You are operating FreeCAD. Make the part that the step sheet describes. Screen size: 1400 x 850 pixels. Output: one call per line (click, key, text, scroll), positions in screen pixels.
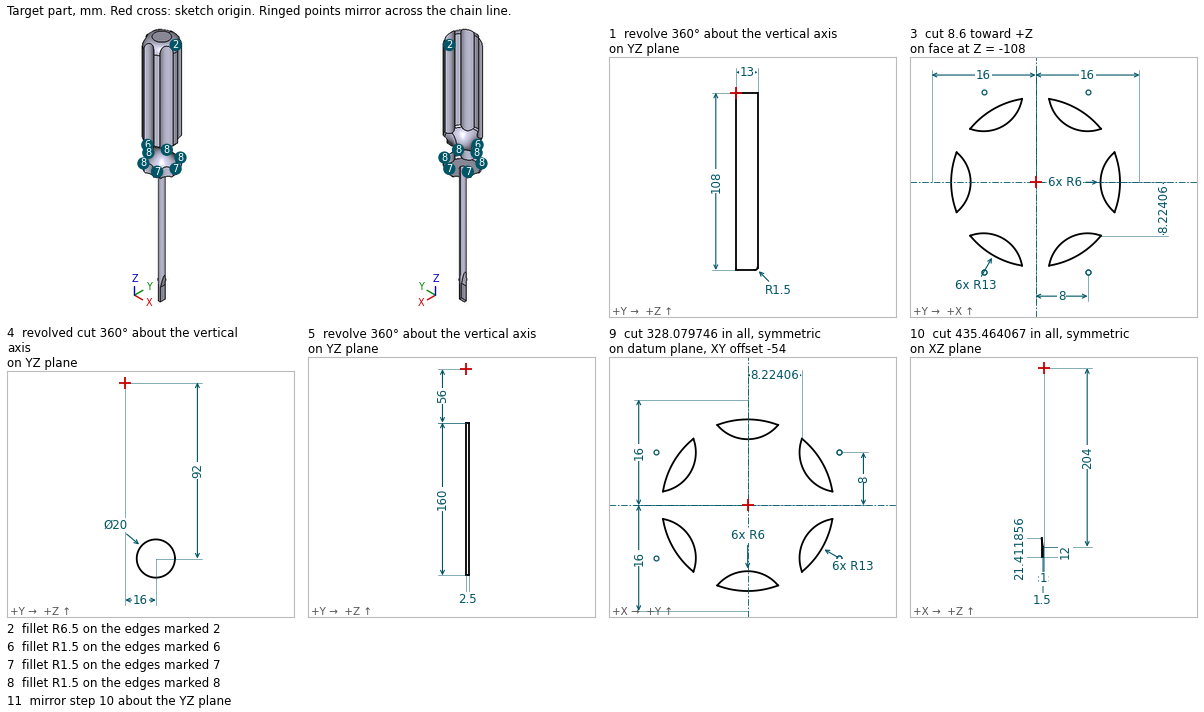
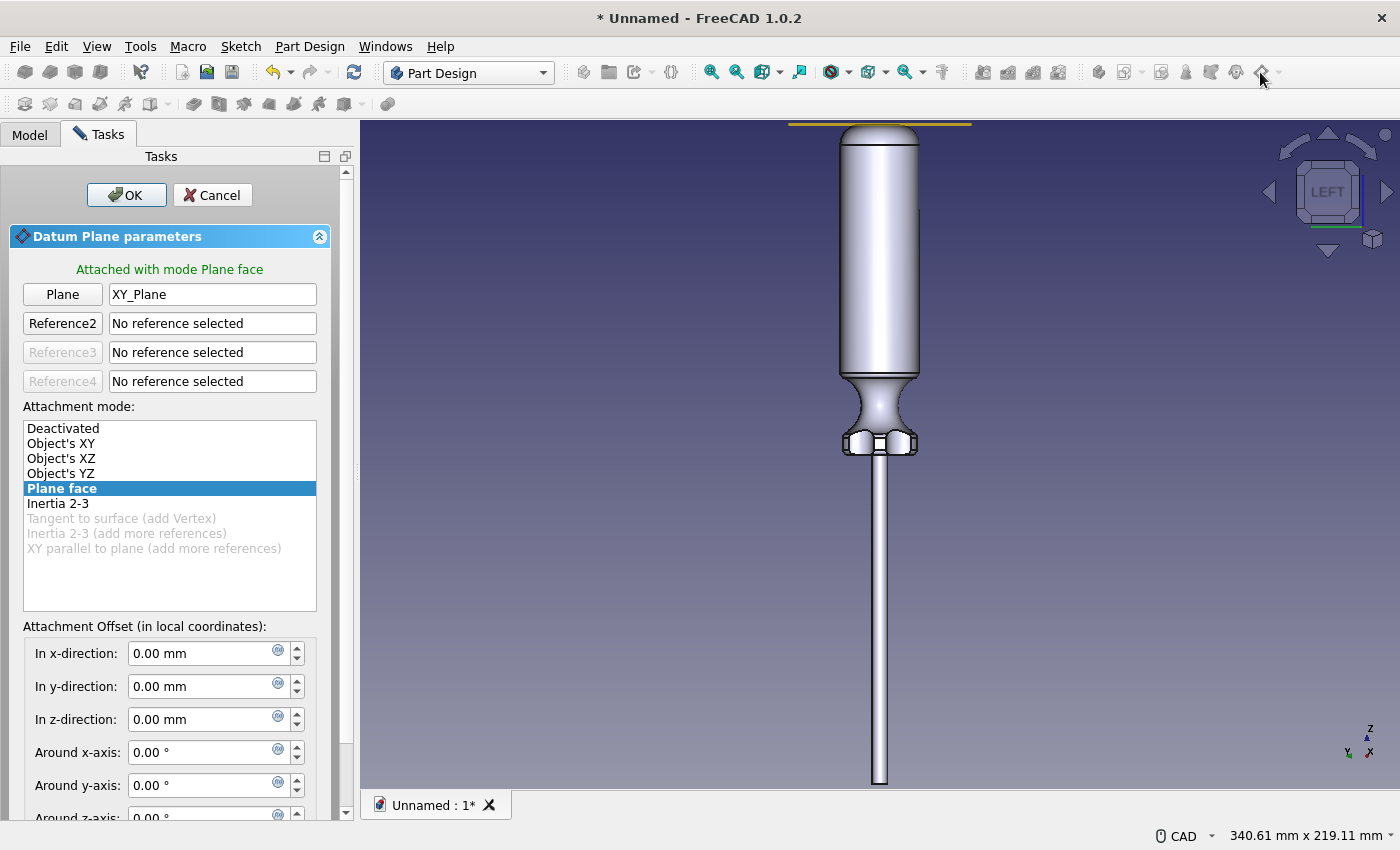
triple_click(210, 720)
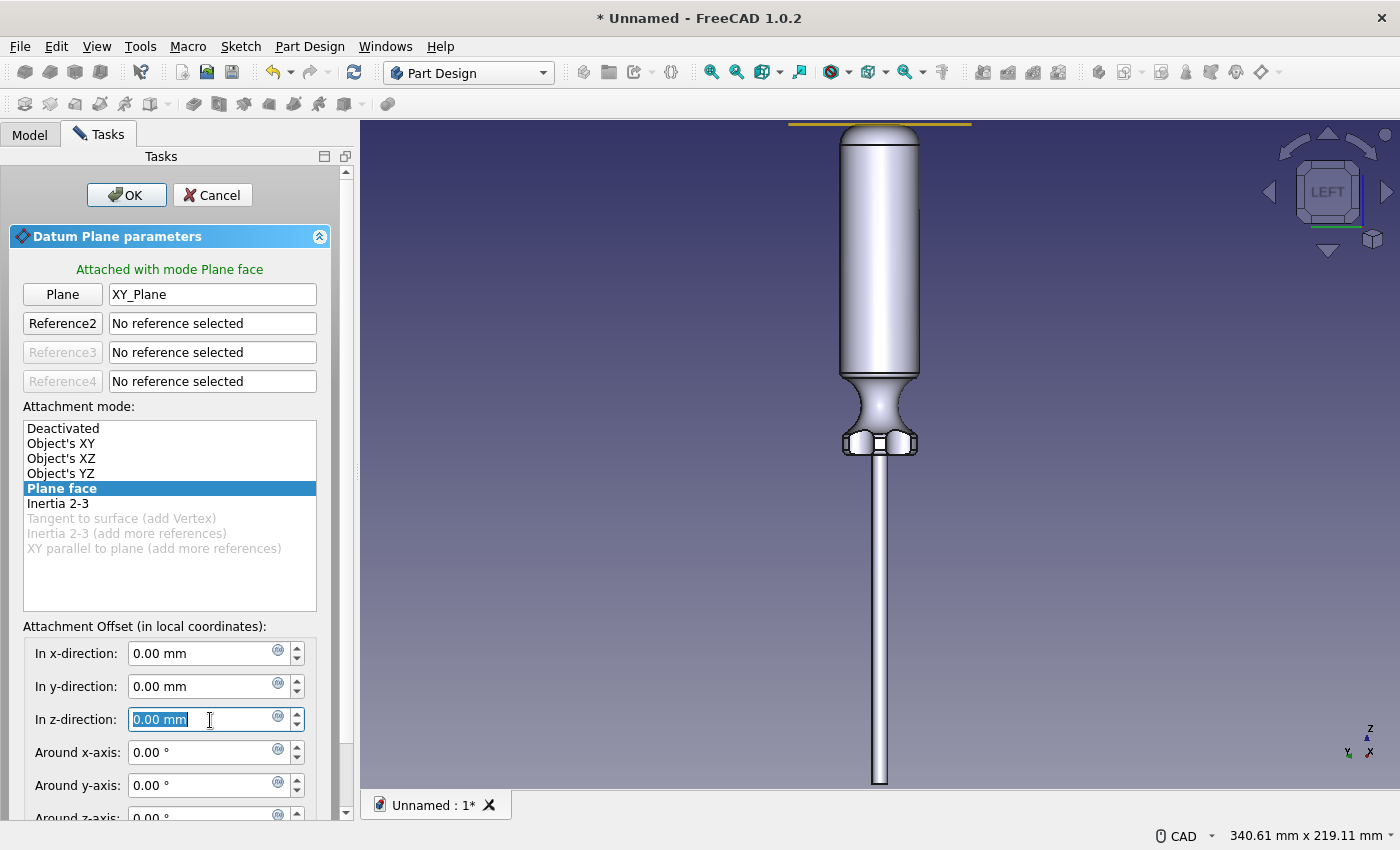
text(-54)
key(Tab)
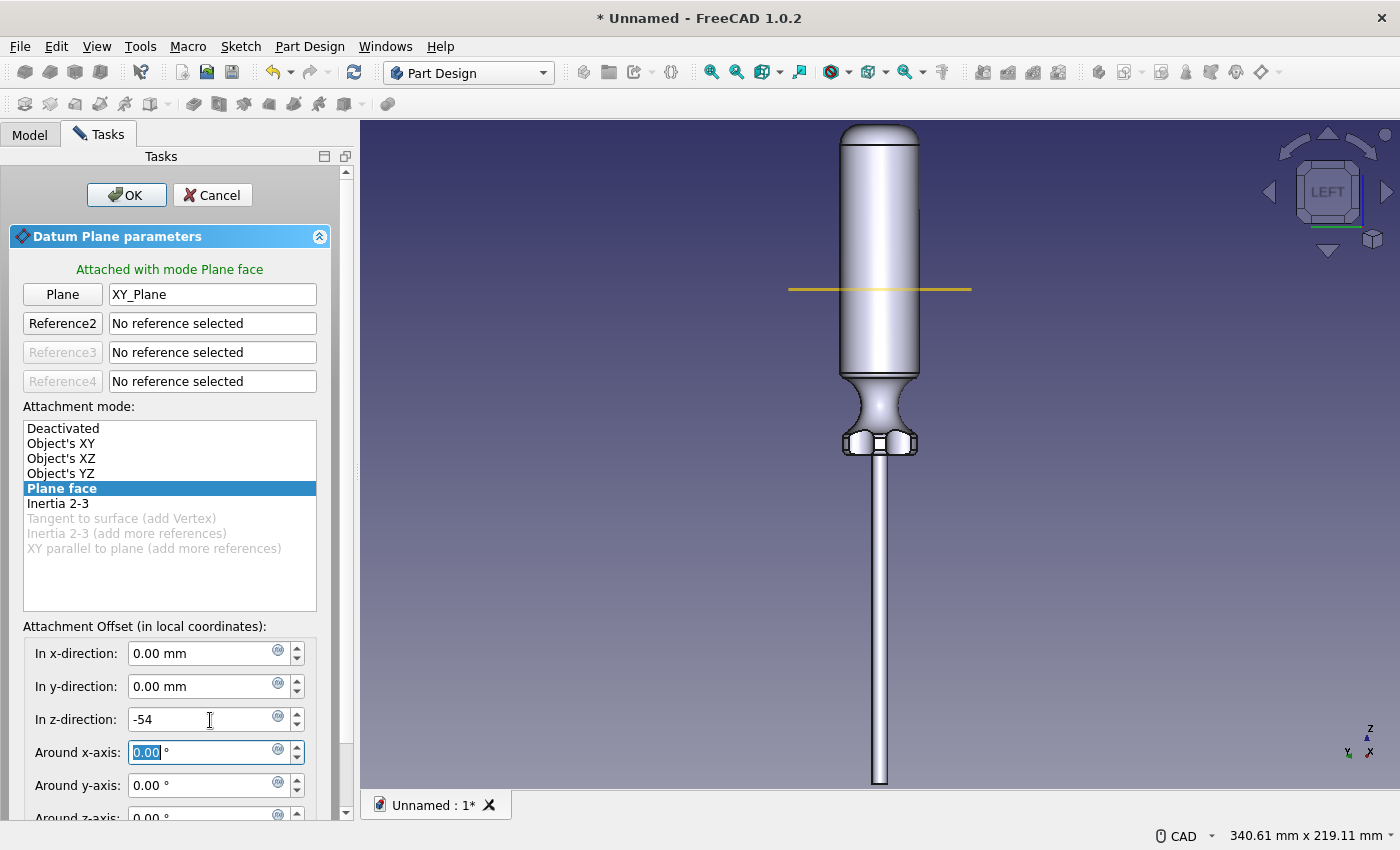
click(127, 195)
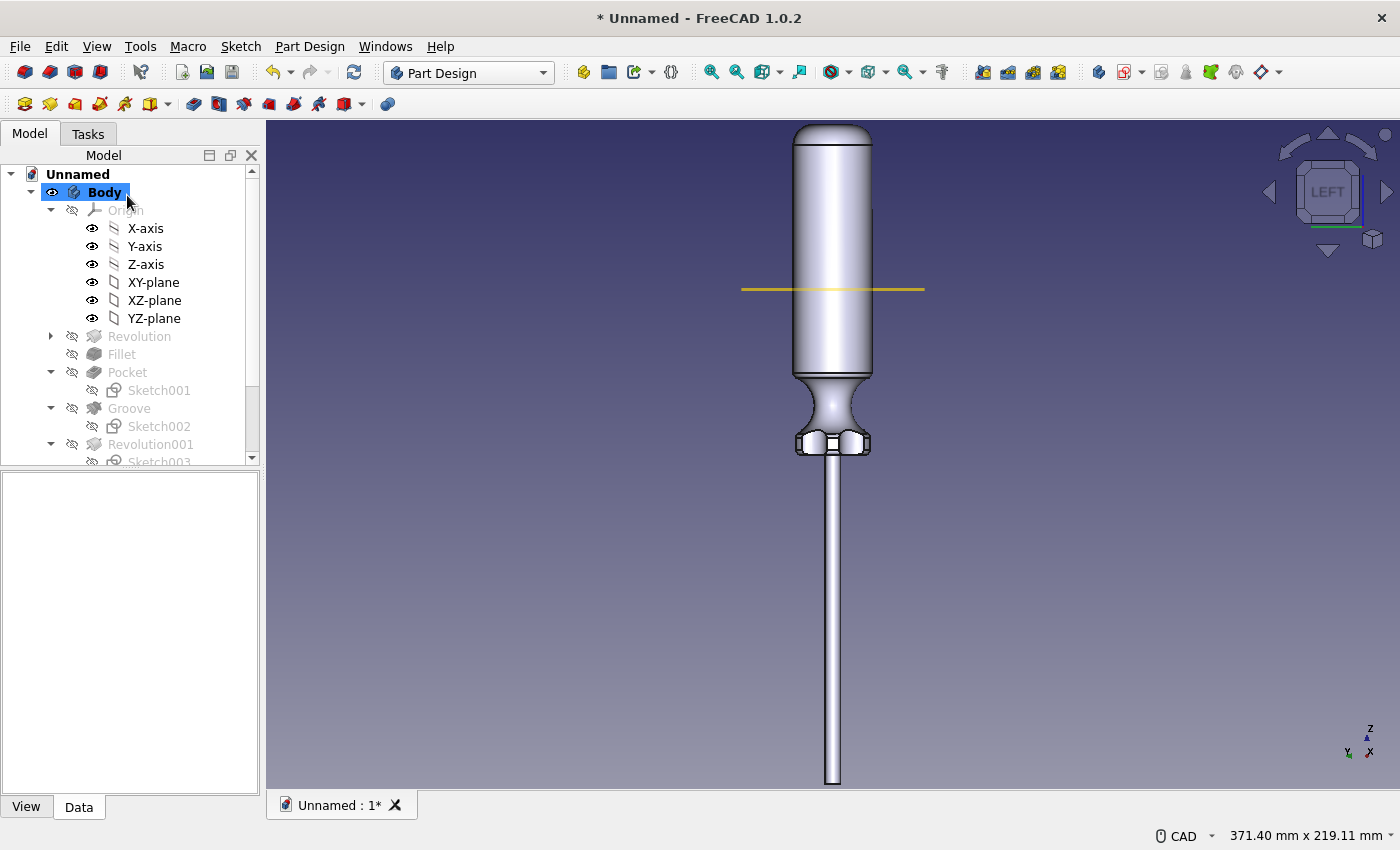
scroll(101, 314, down, 3)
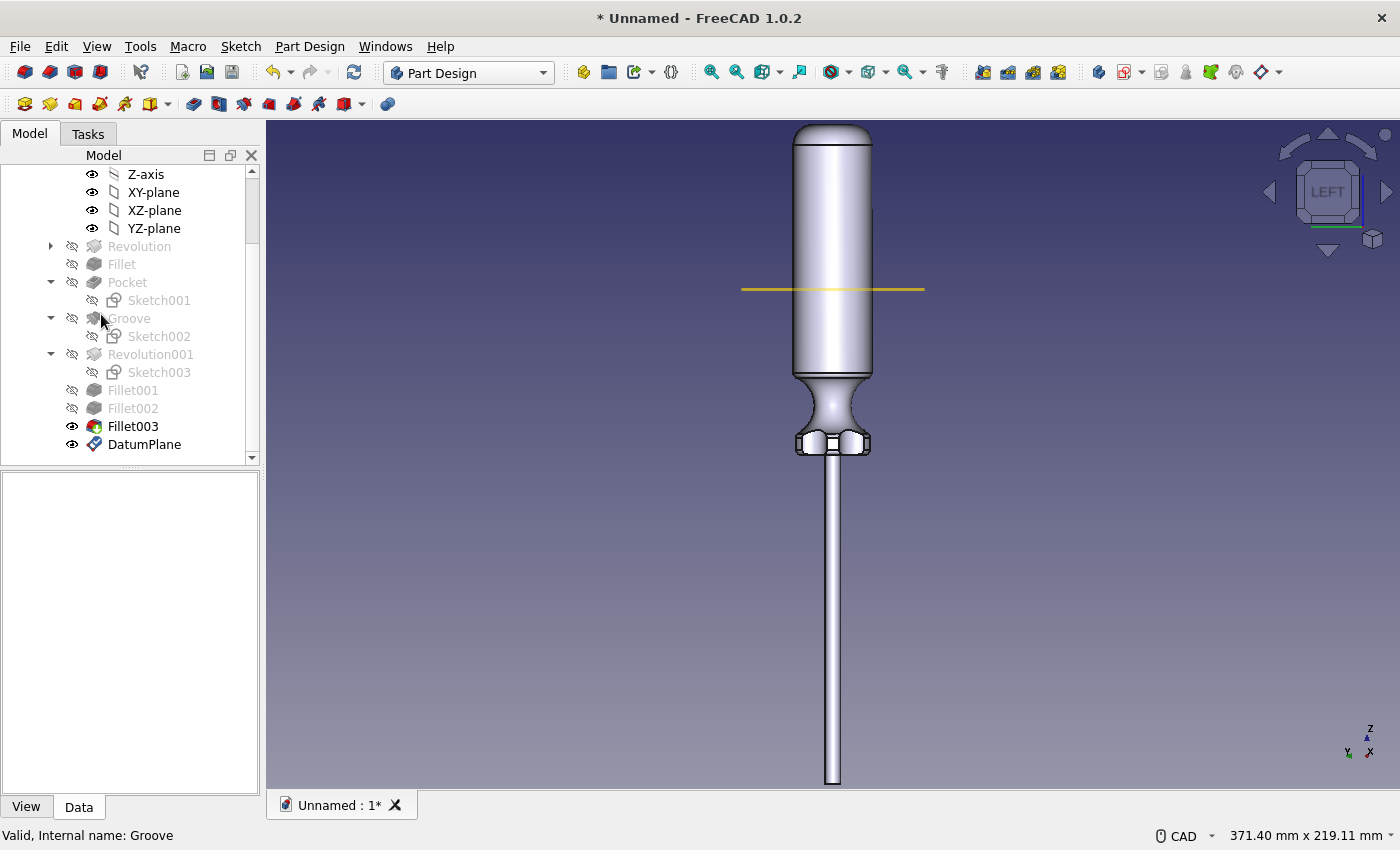
click(117, 444)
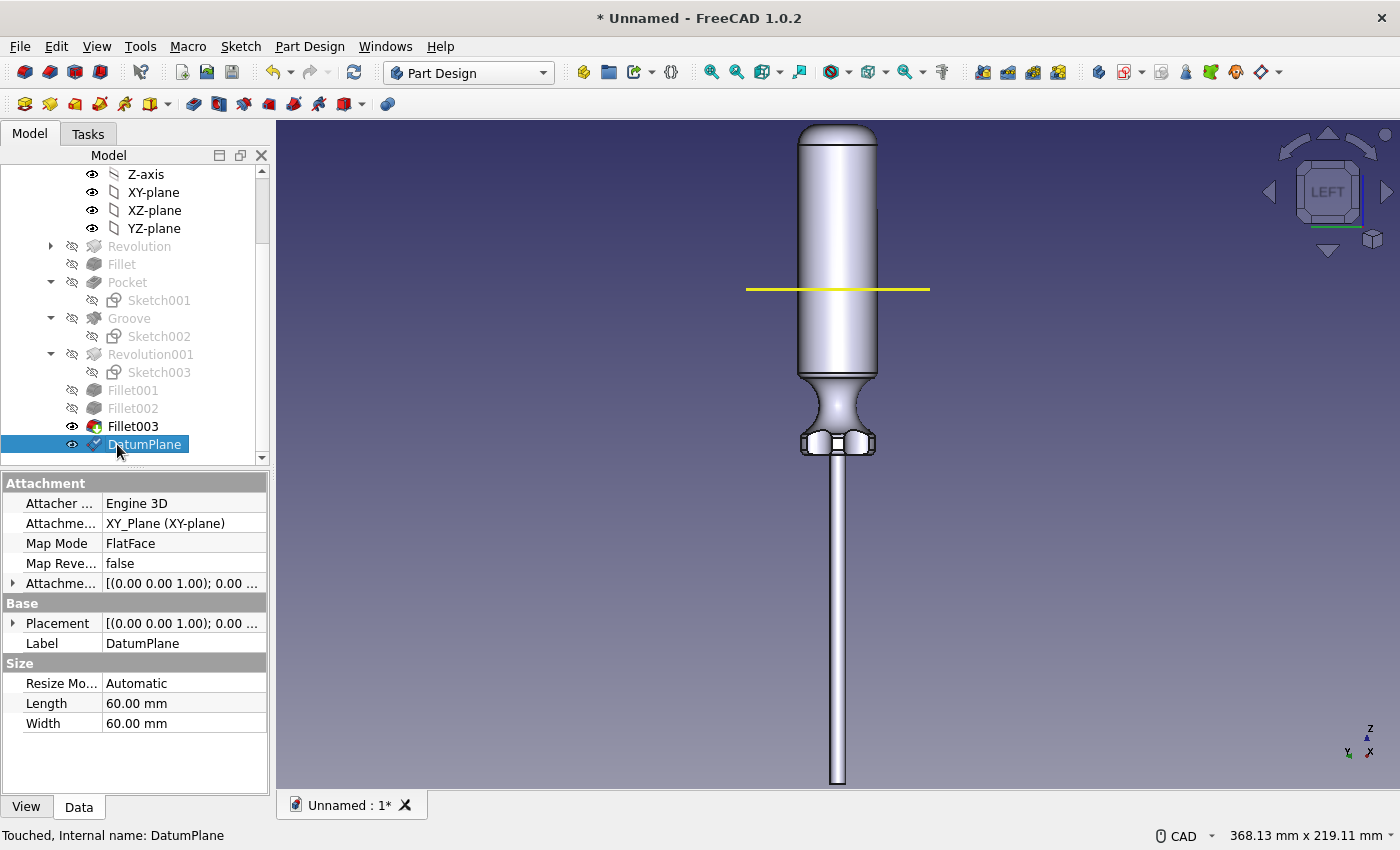
click(1124, 72)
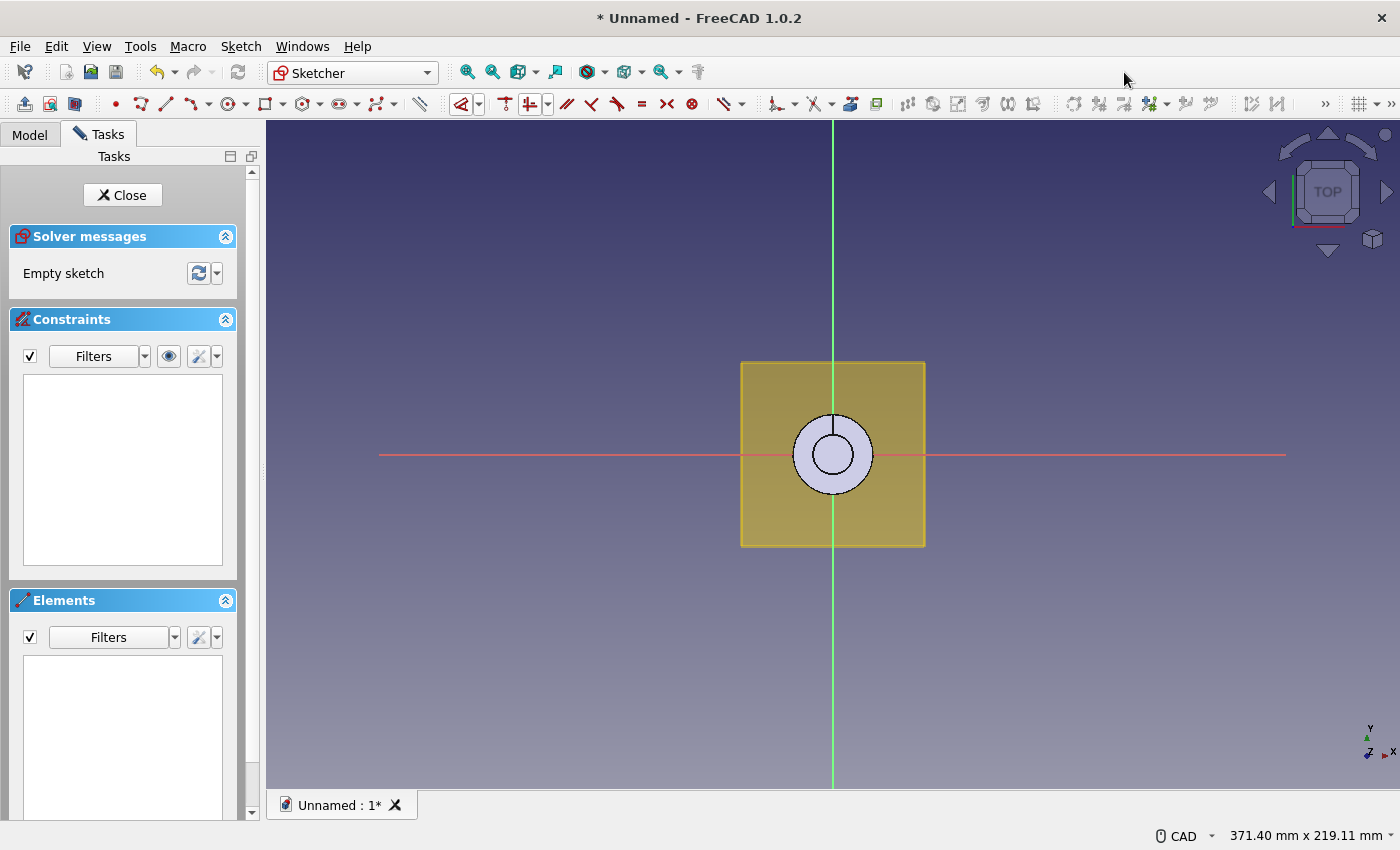
click(75, 104)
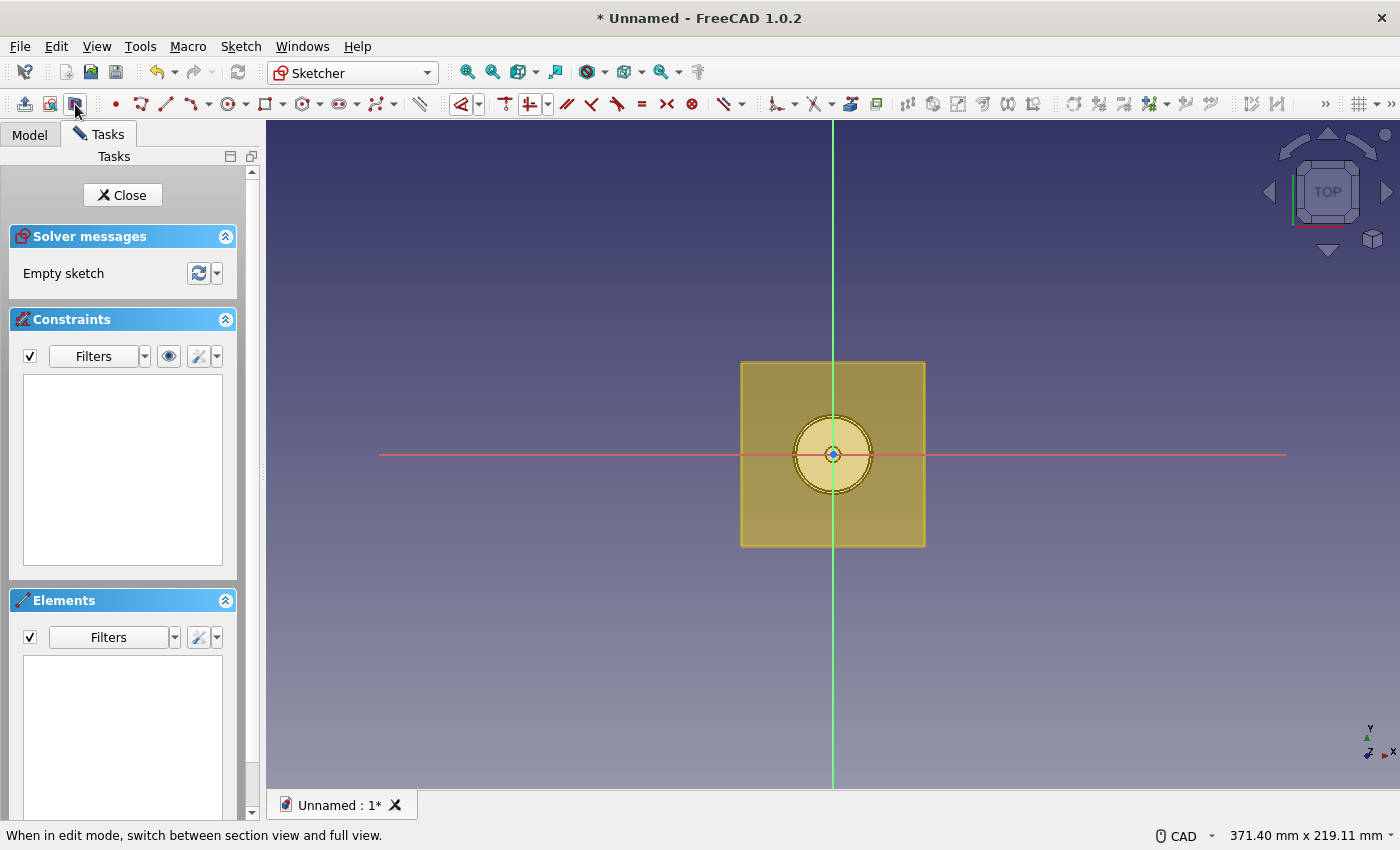
scroll(850, 455, up, 8)